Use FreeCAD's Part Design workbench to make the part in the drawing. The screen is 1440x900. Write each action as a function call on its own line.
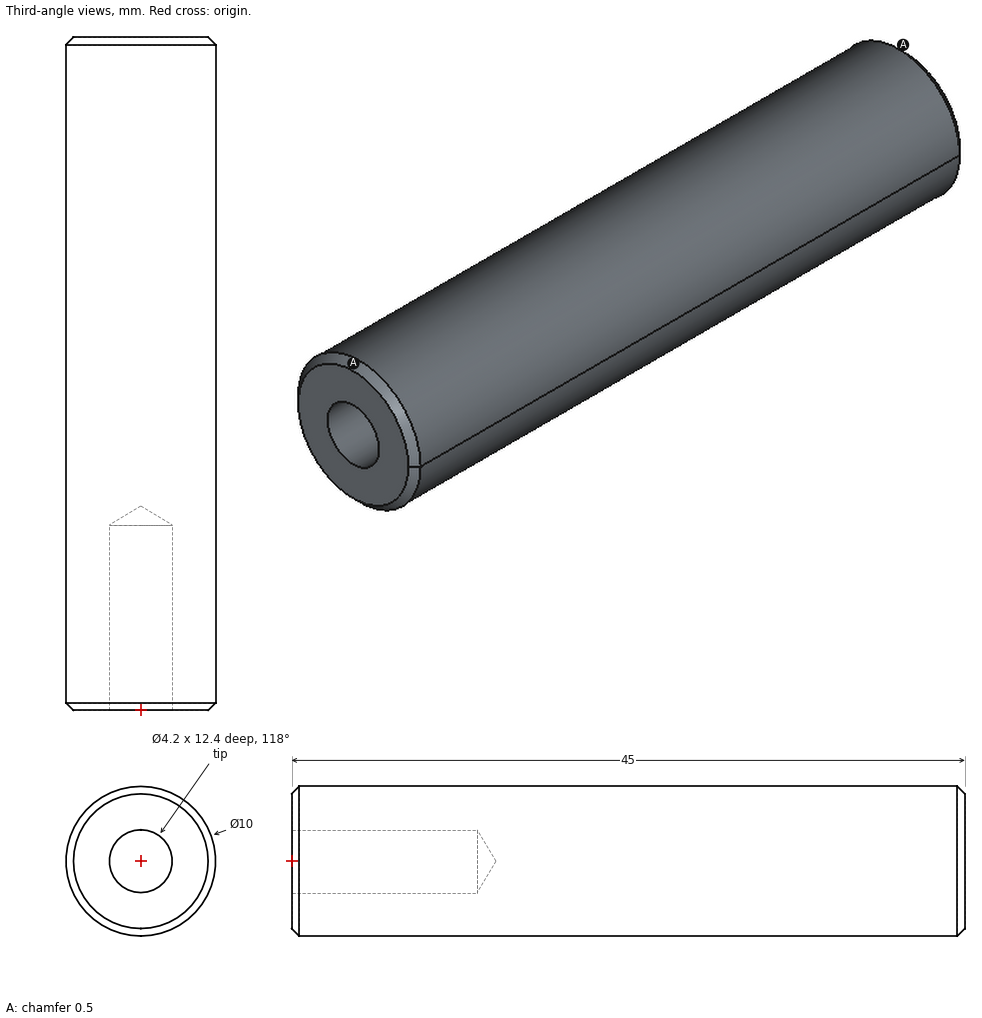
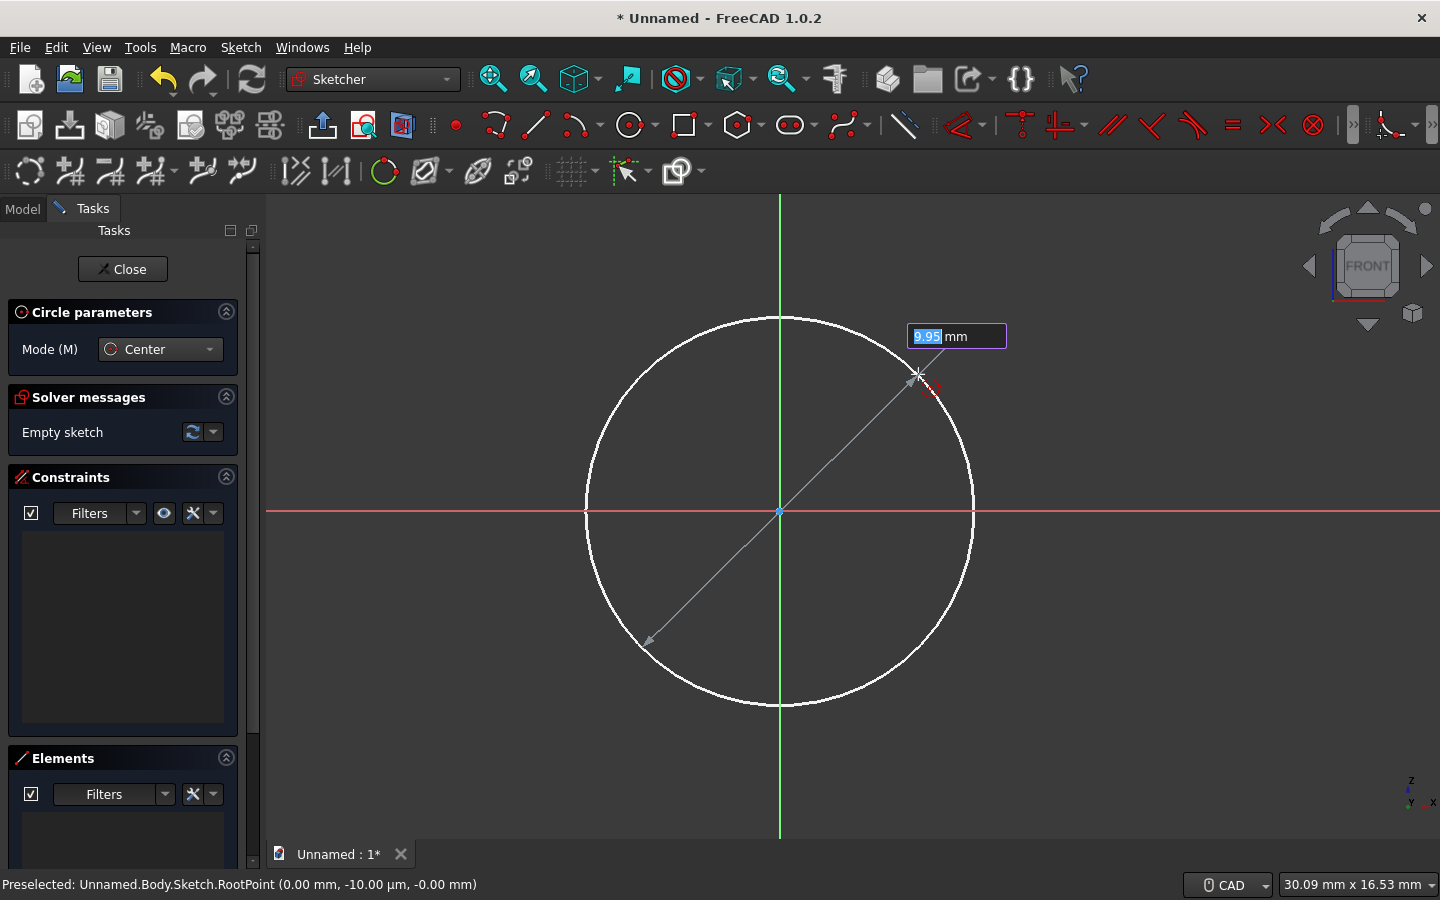
text(10)
key(Return)
key(Escape)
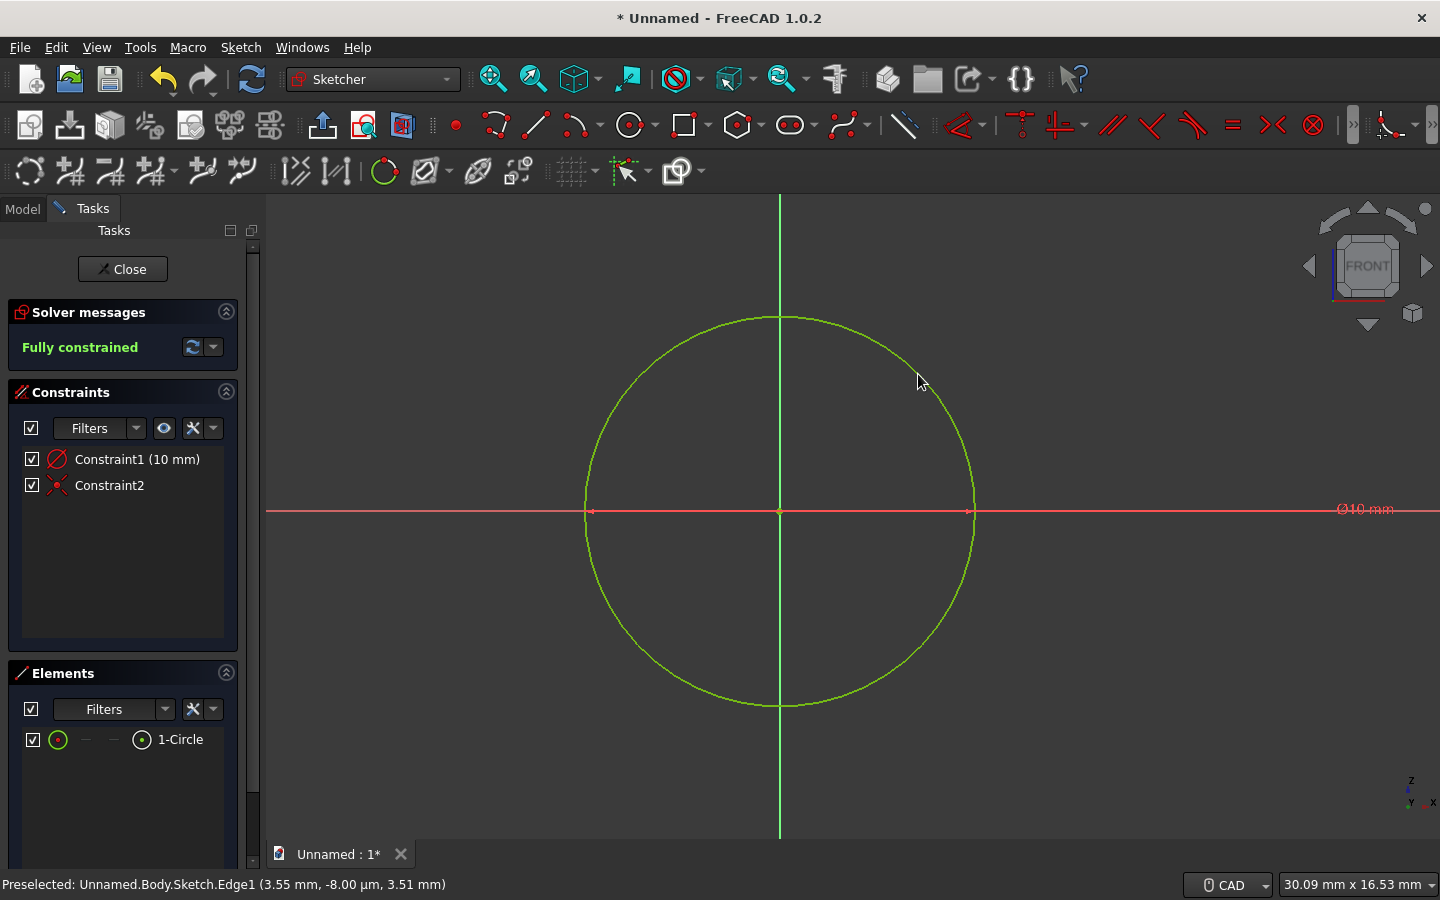
click(123, 269)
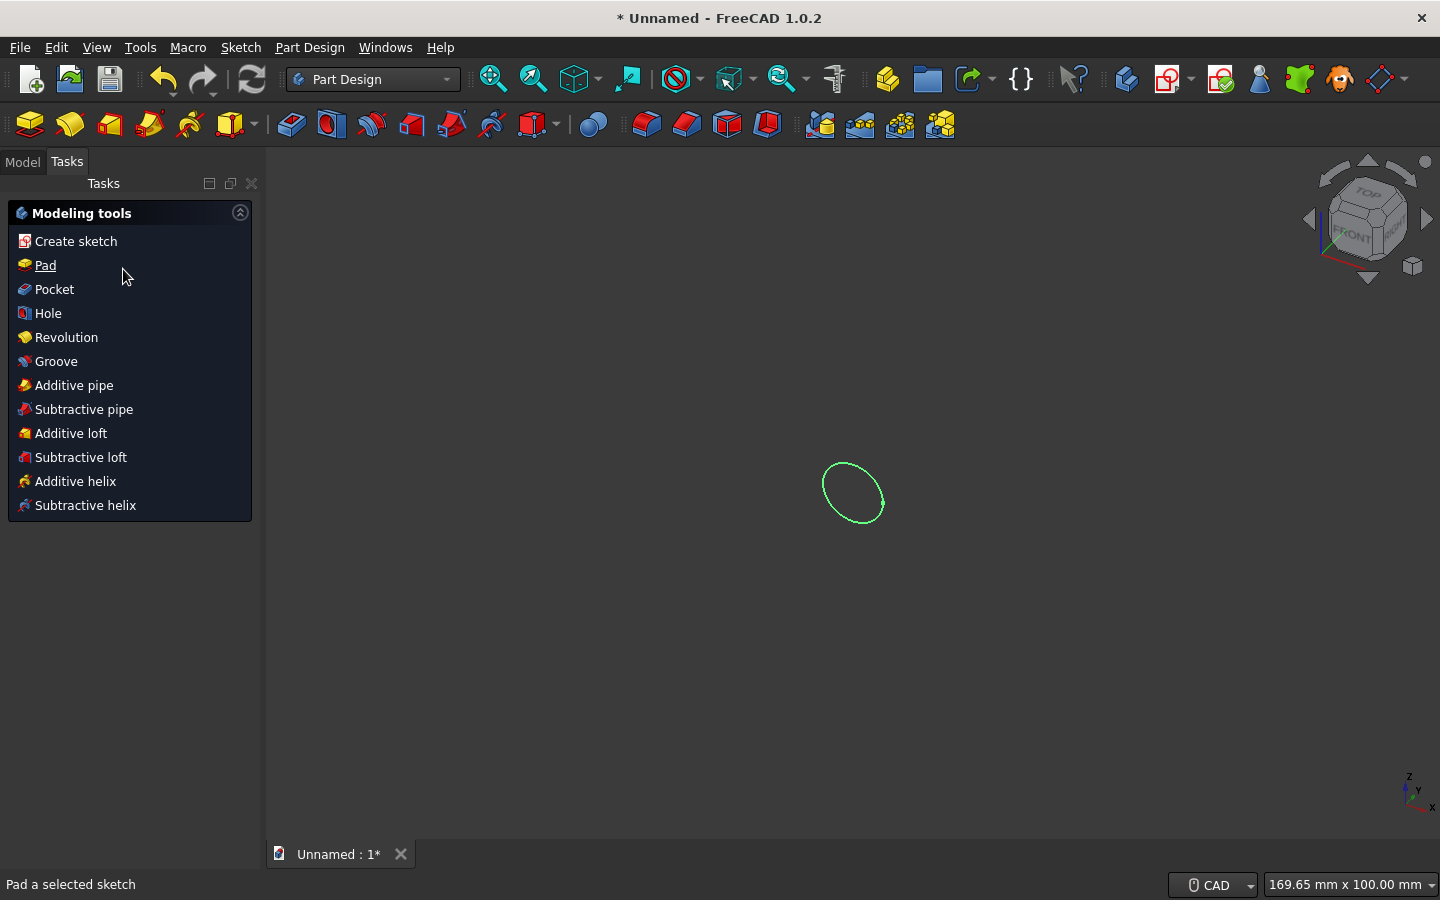
click(30, 124)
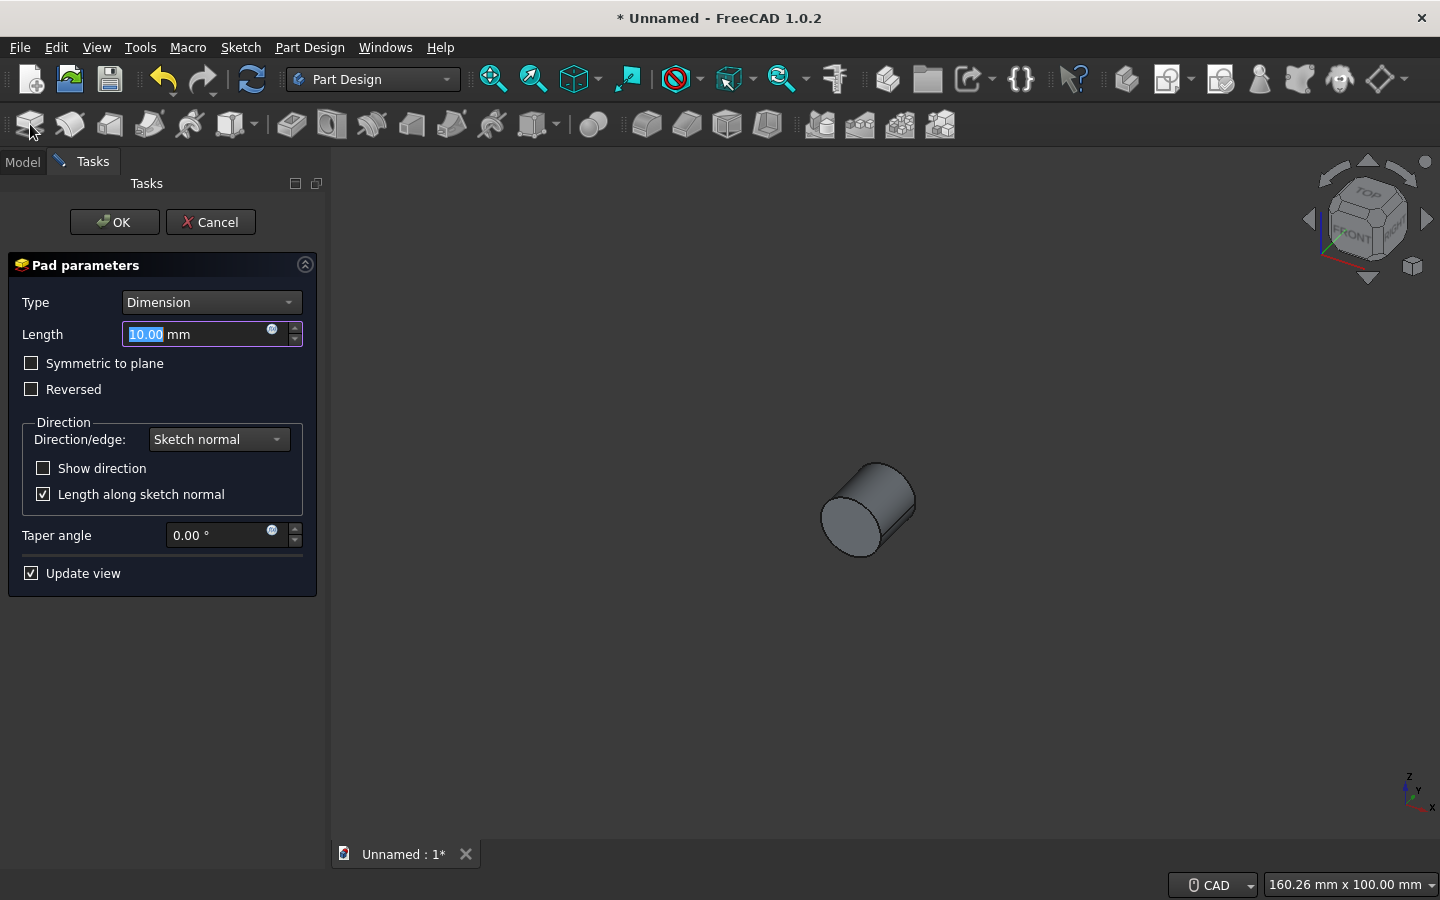
text(45)
key(Tab)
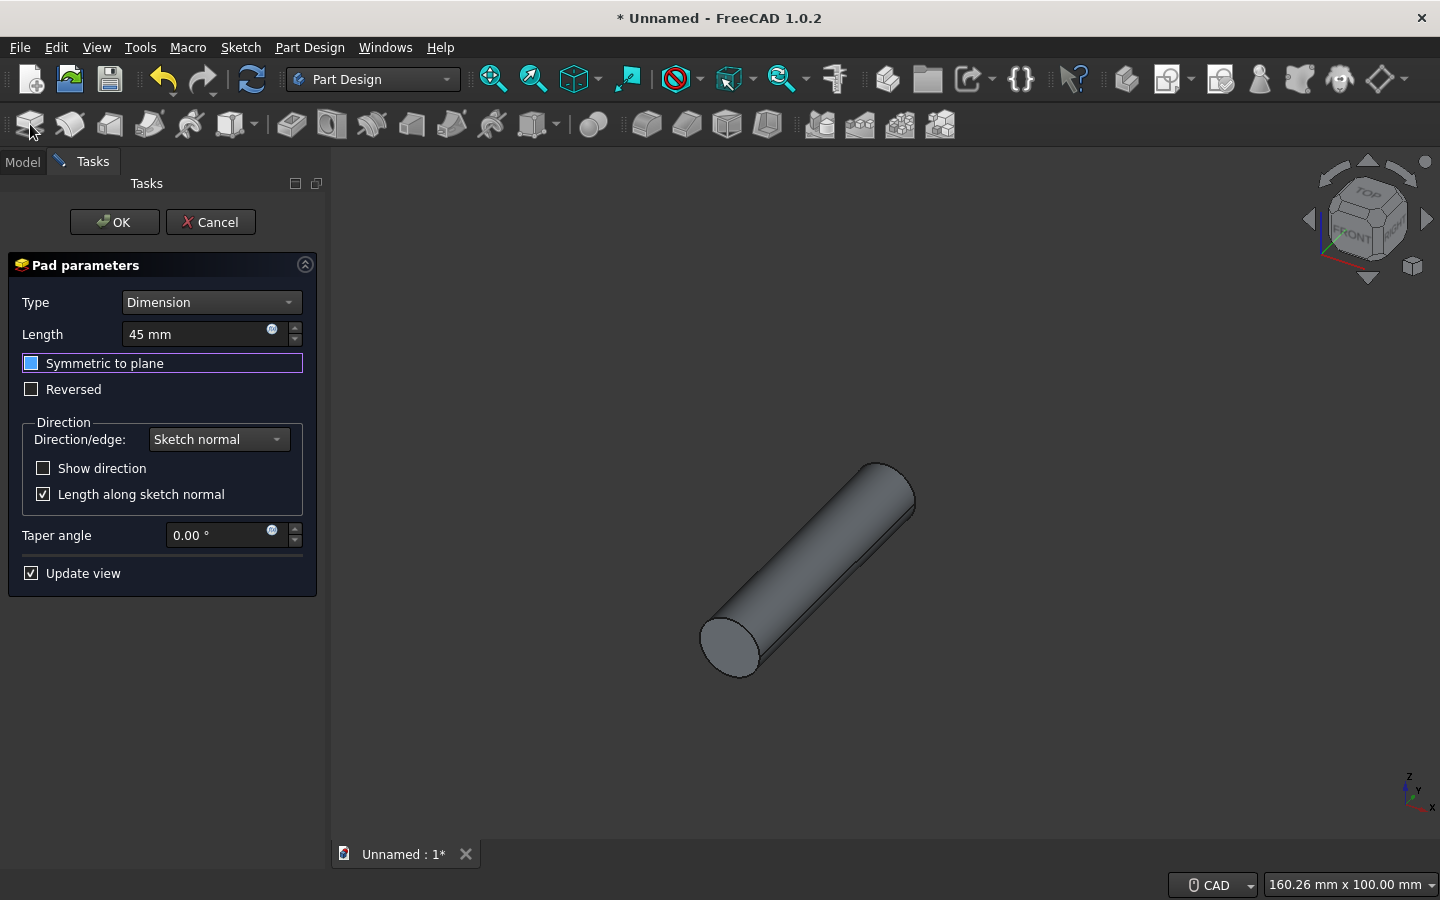
click(30, 389)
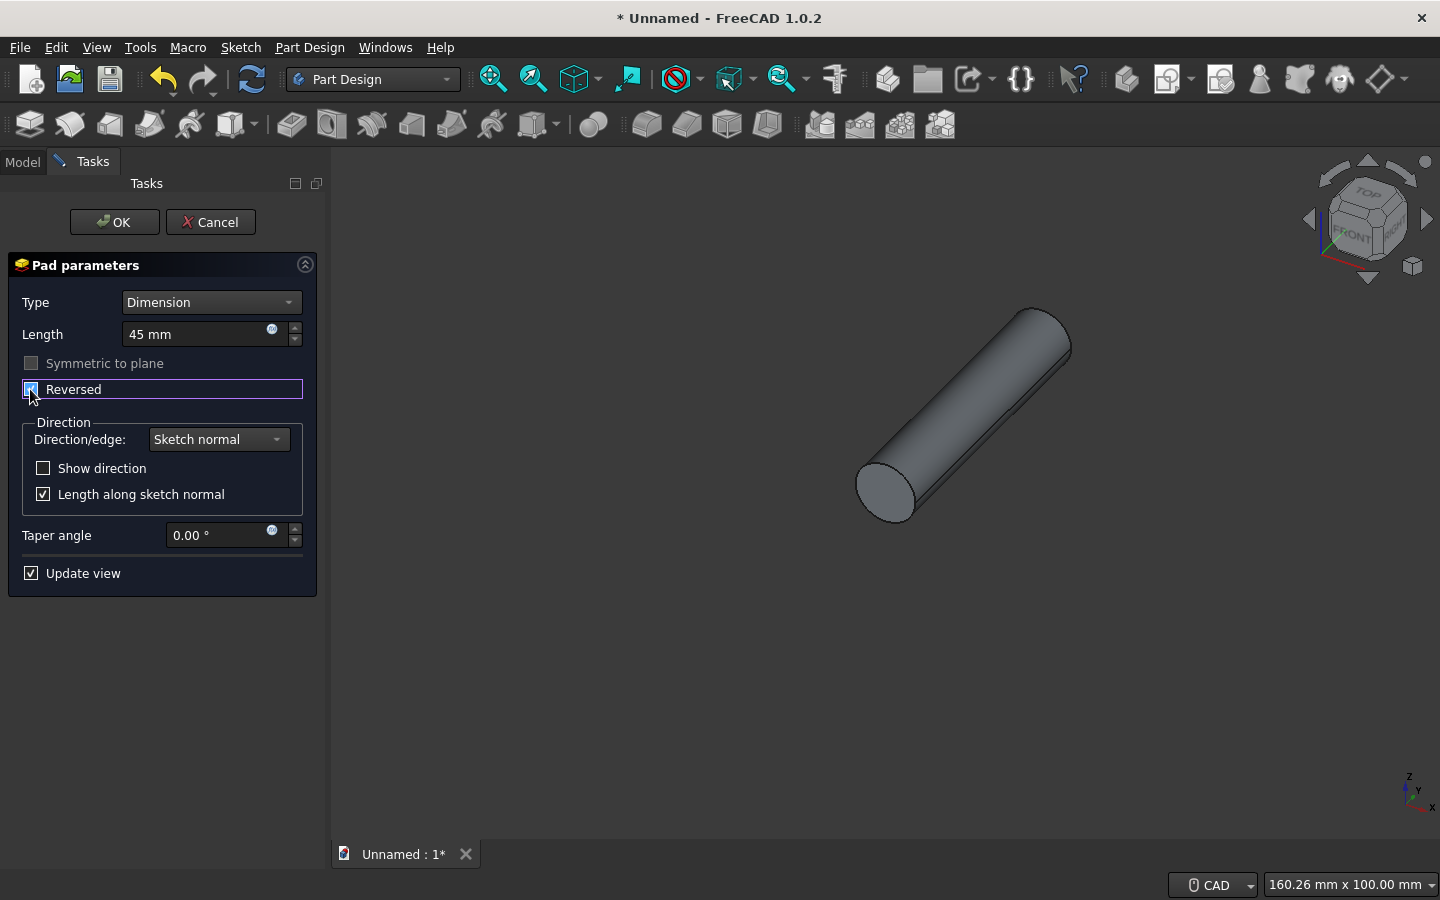
click(115, 222)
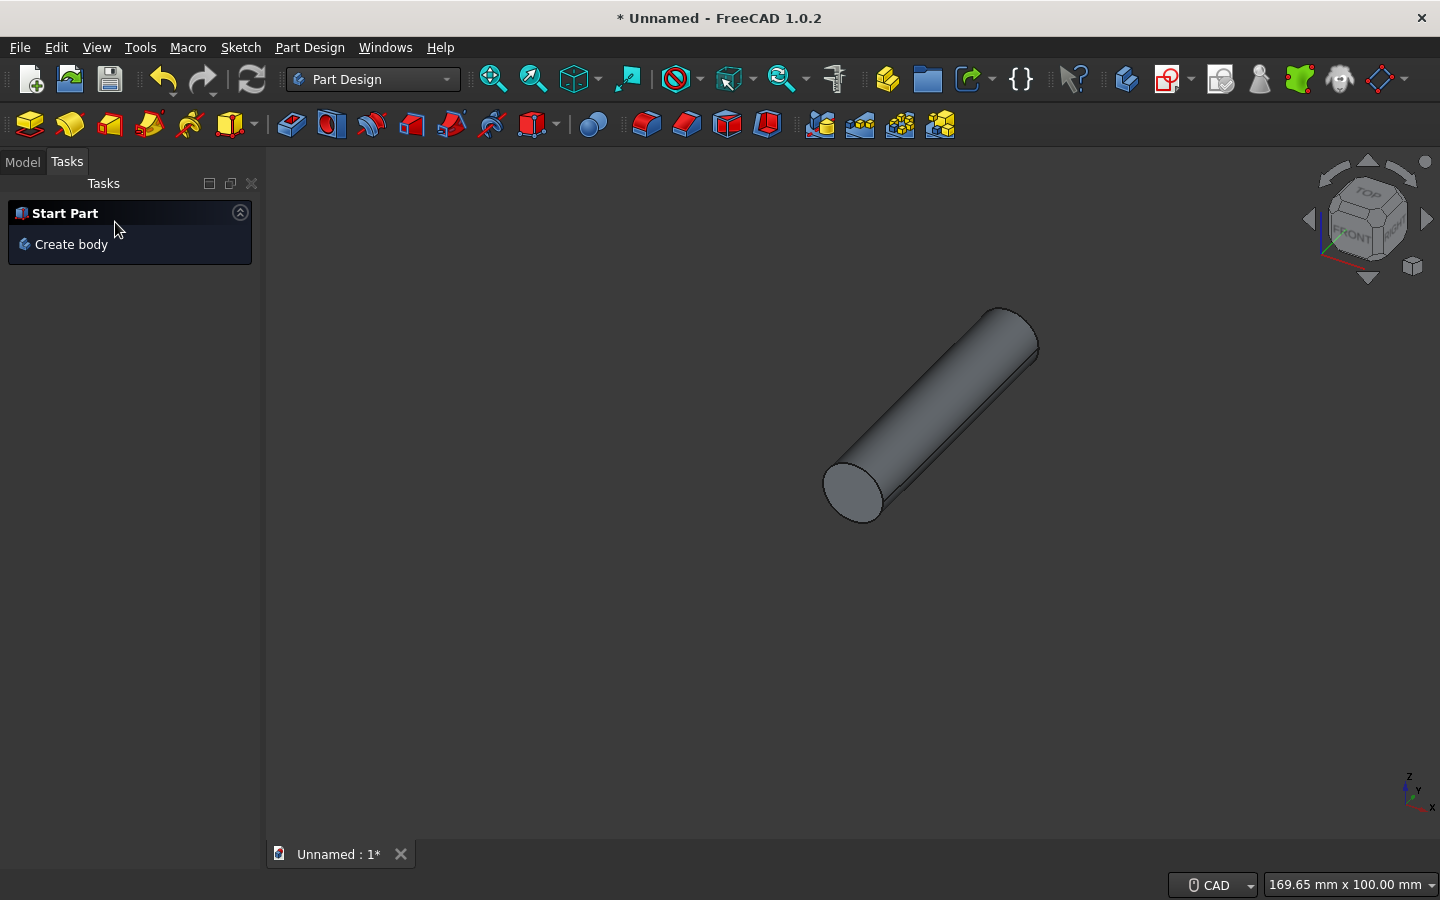
click(494, 80)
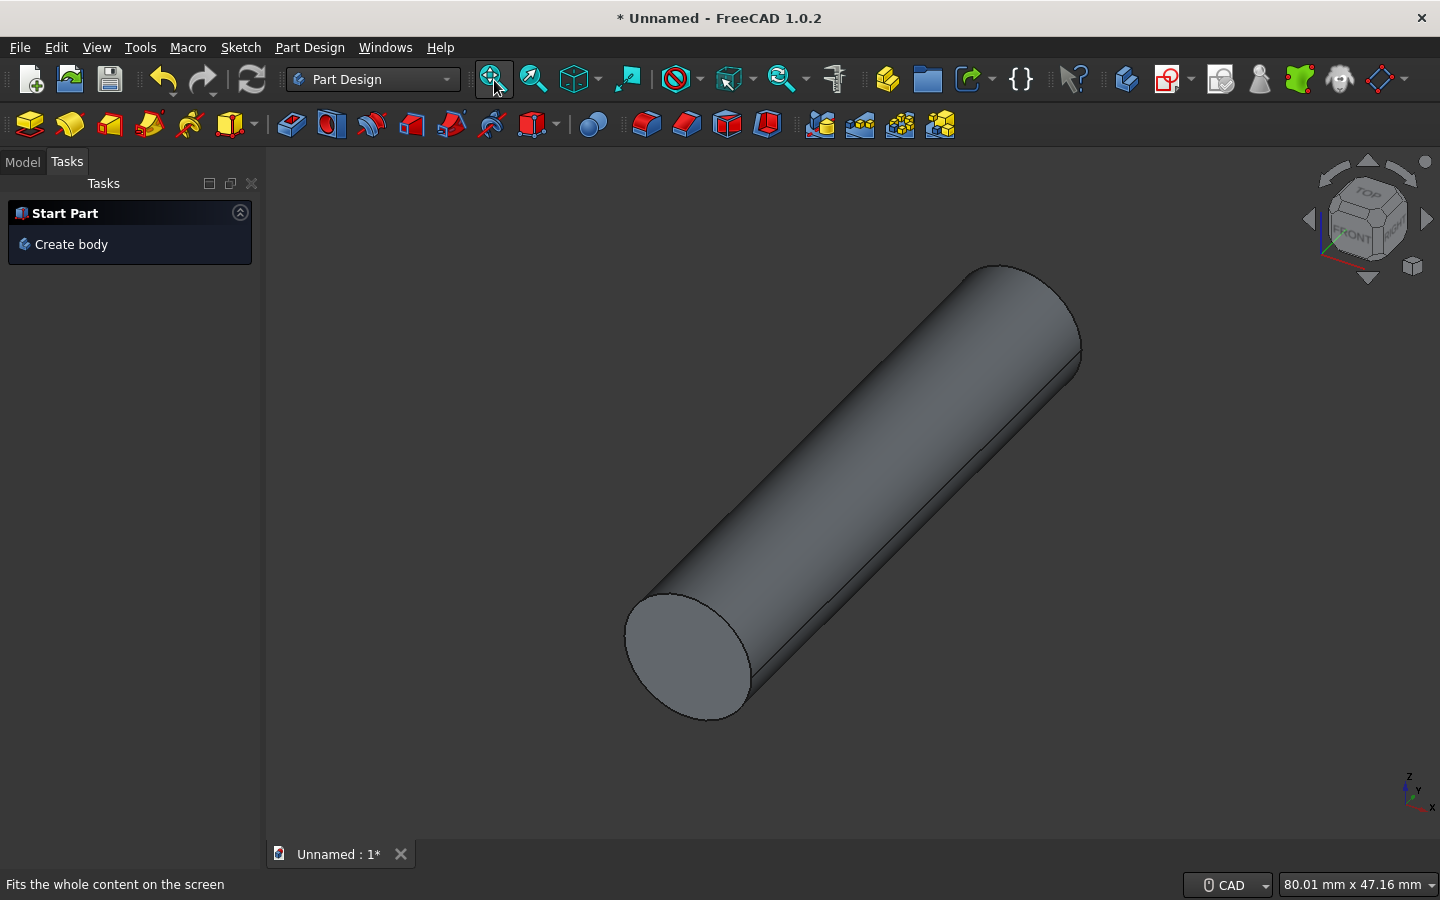
click(688, 656)